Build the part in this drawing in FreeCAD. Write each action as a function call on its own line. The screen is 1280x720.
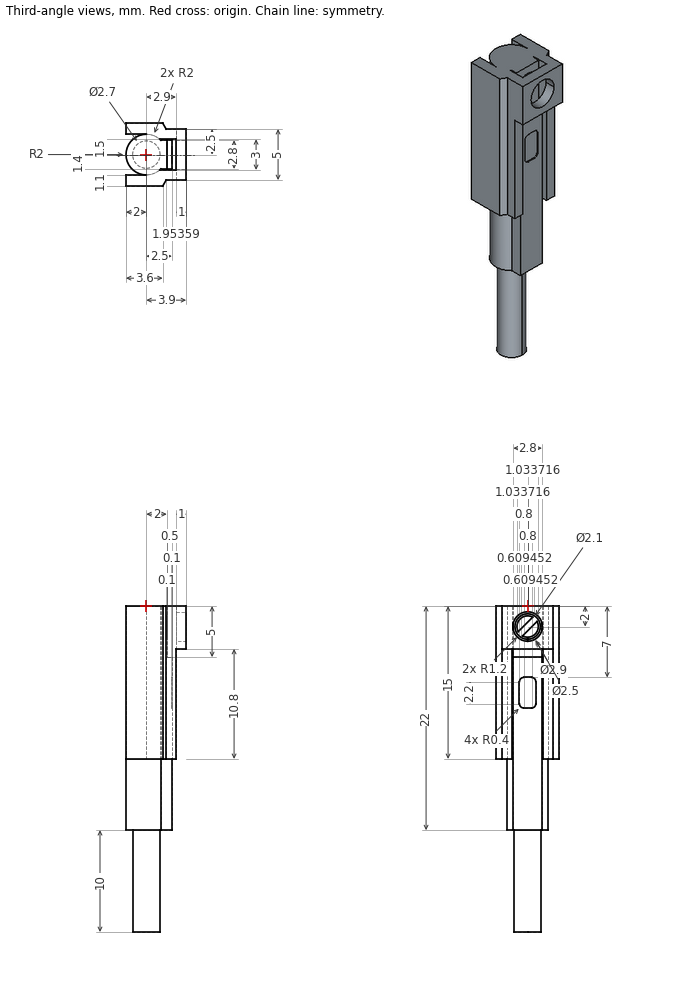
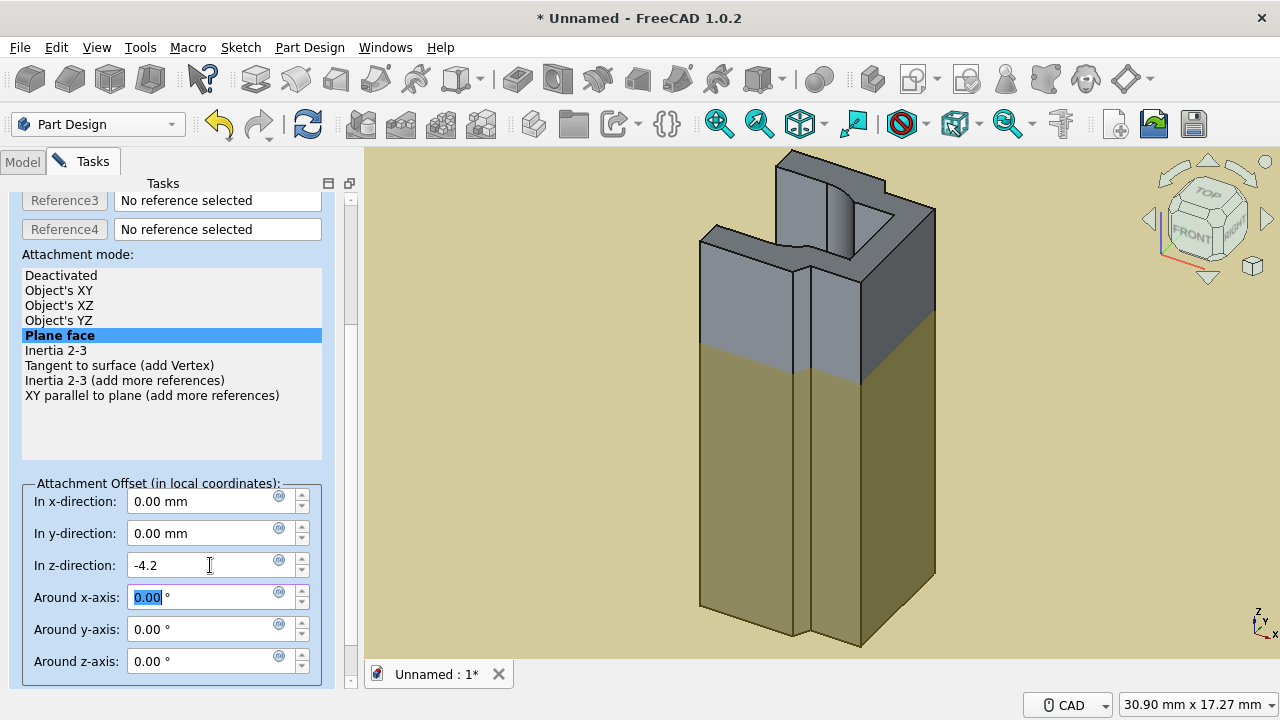
scroll(351, 440, up, 4)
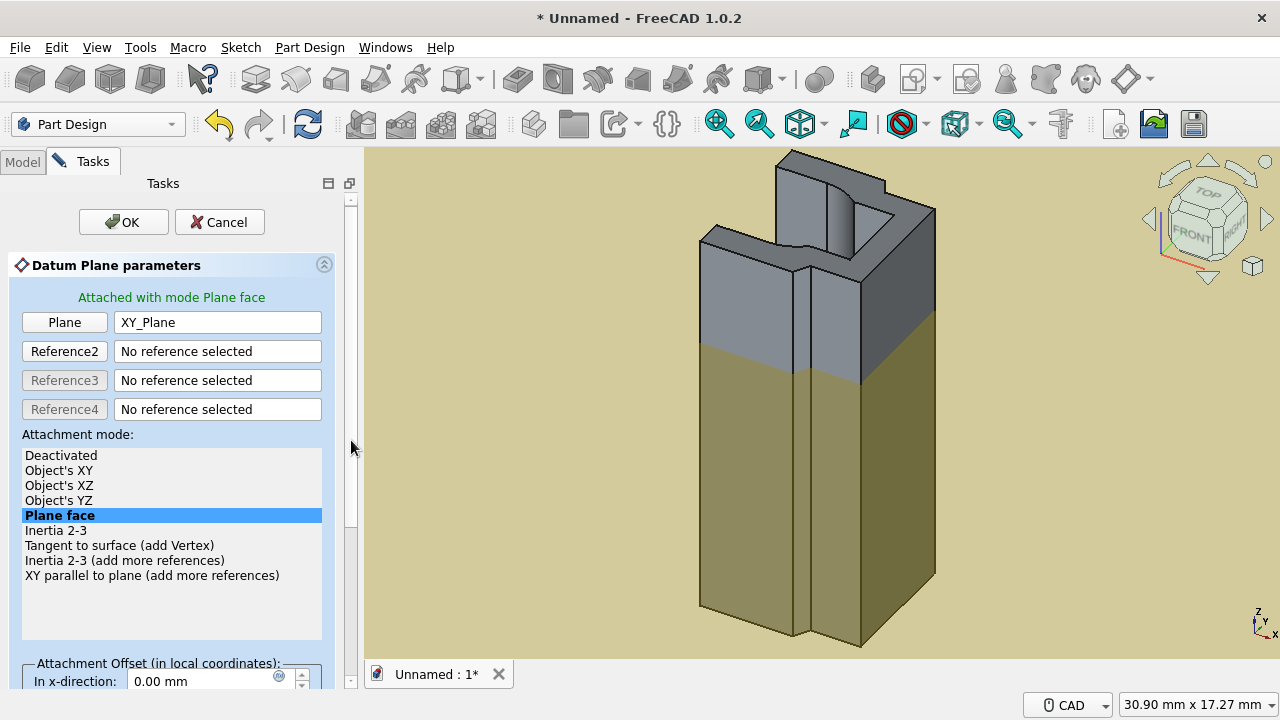
click(124, 222)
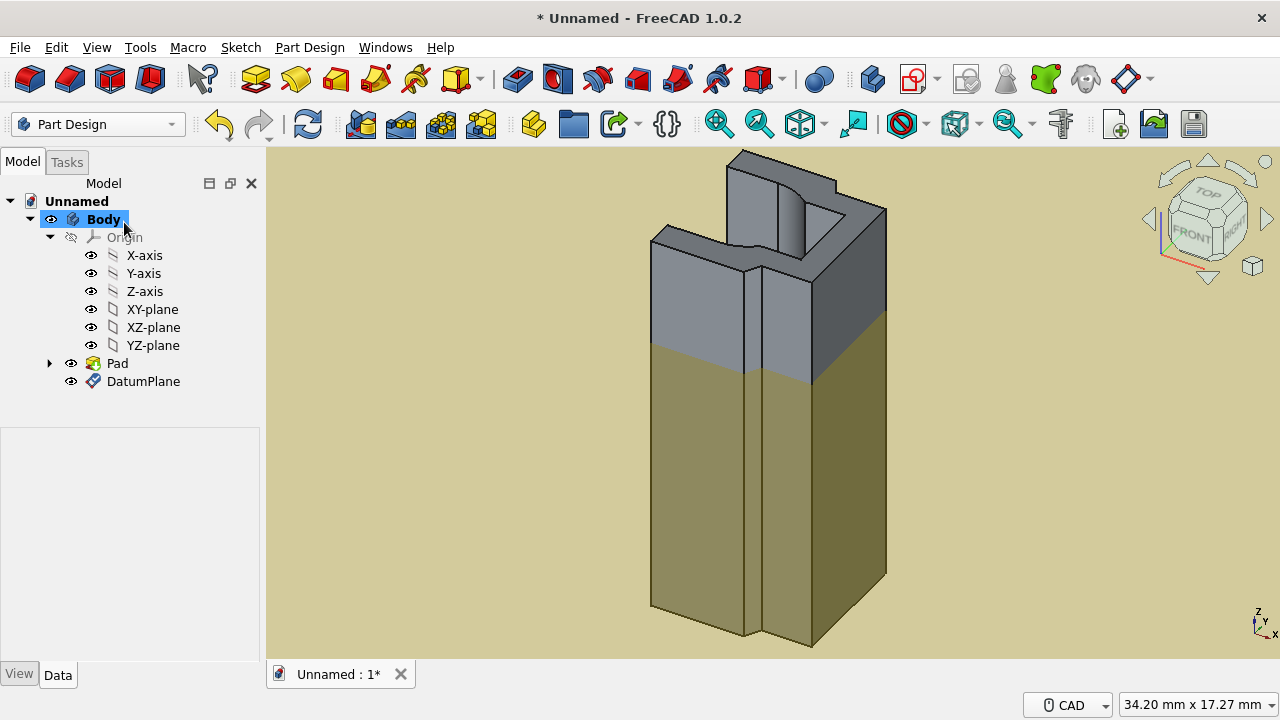
click(116, 381)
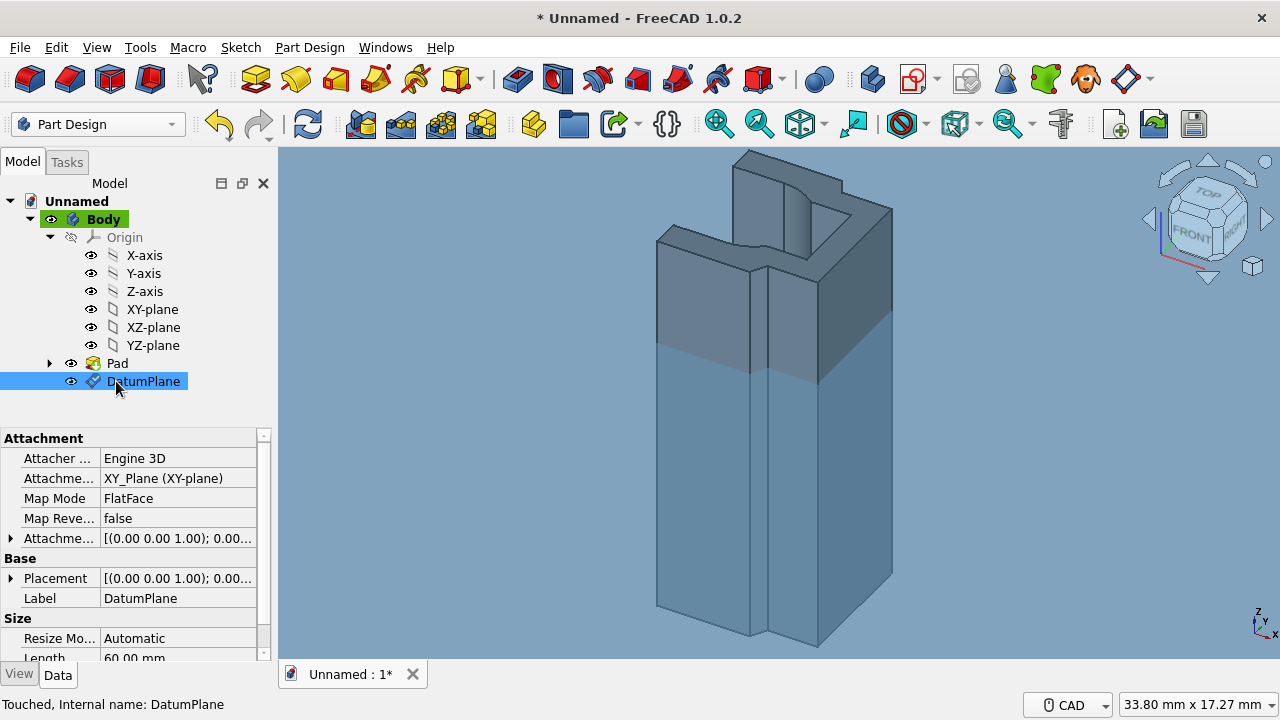
click(914, 80)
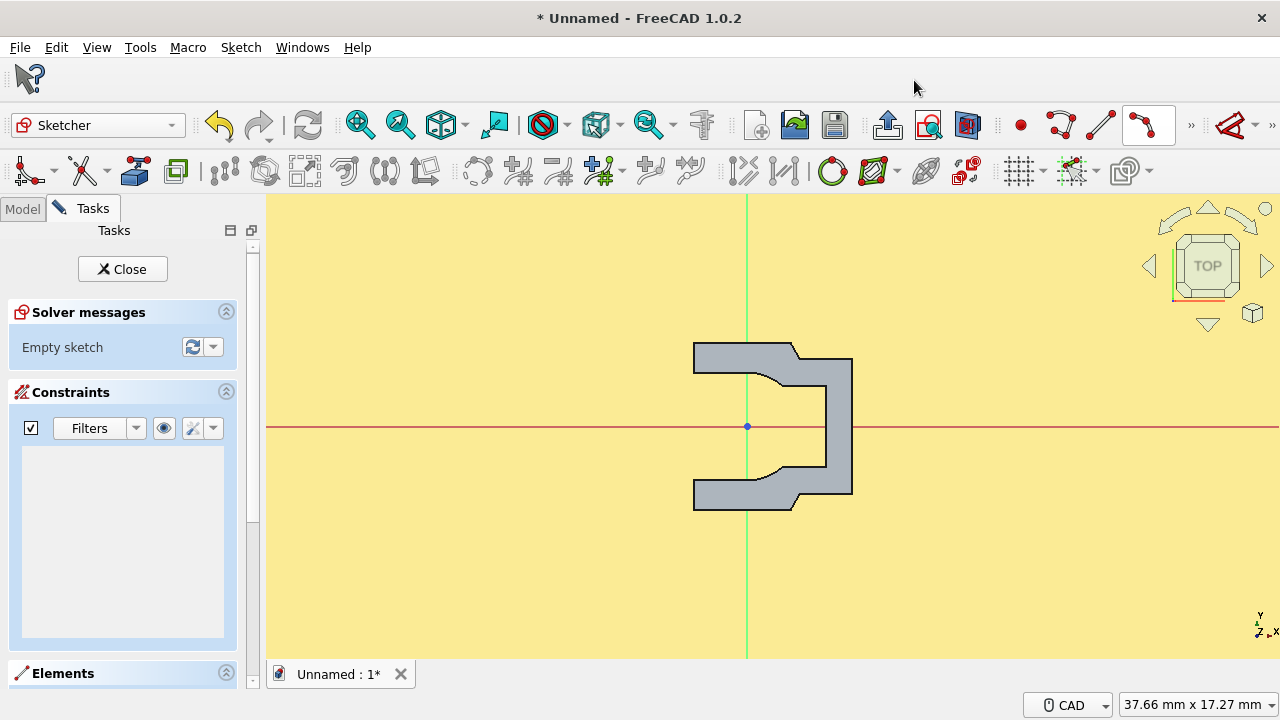
click(968, 126)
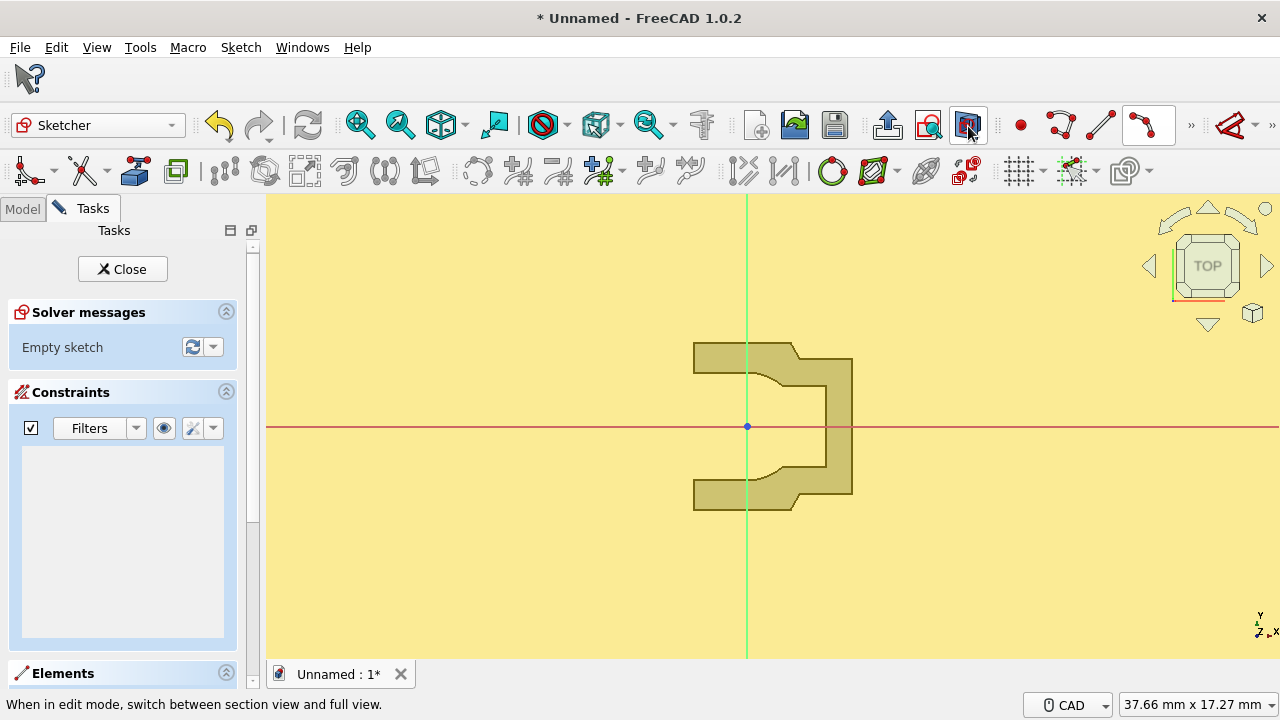
scroll(878, 426, up, 4)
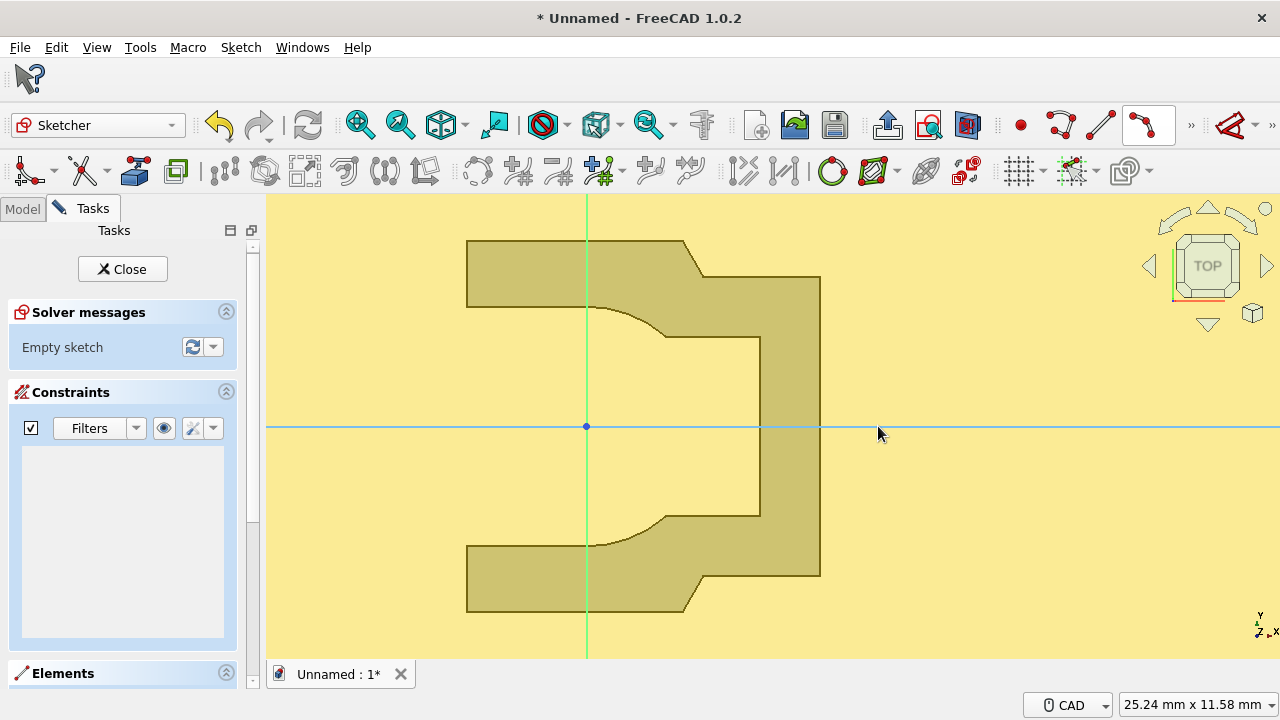
key(g)
key(r)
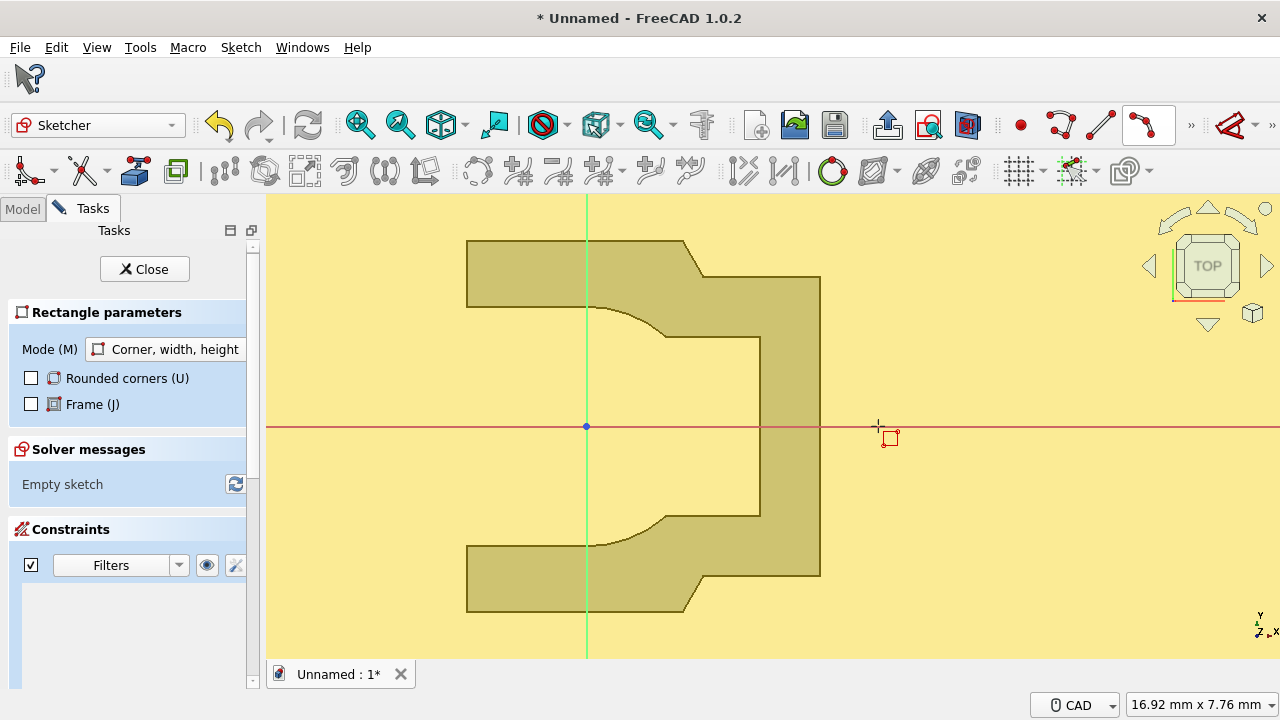
click(760, 277)
click(820, 576)
key(Escape)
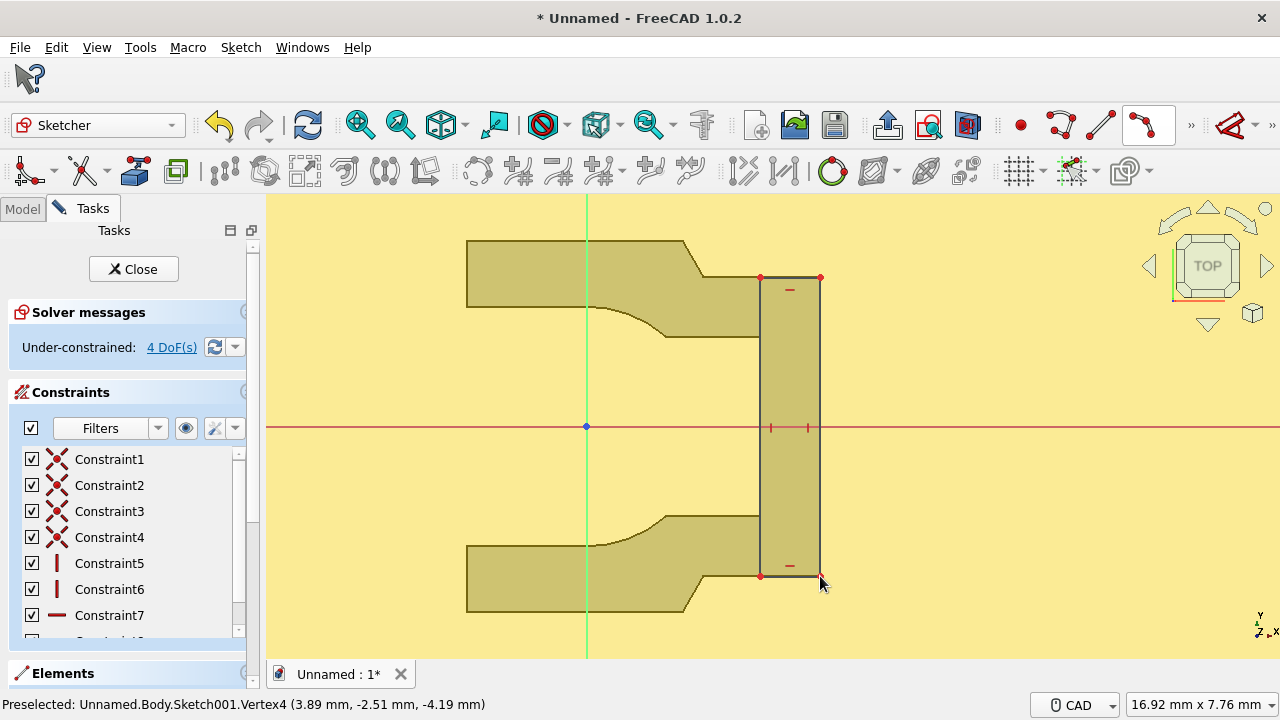
click(1230, 126)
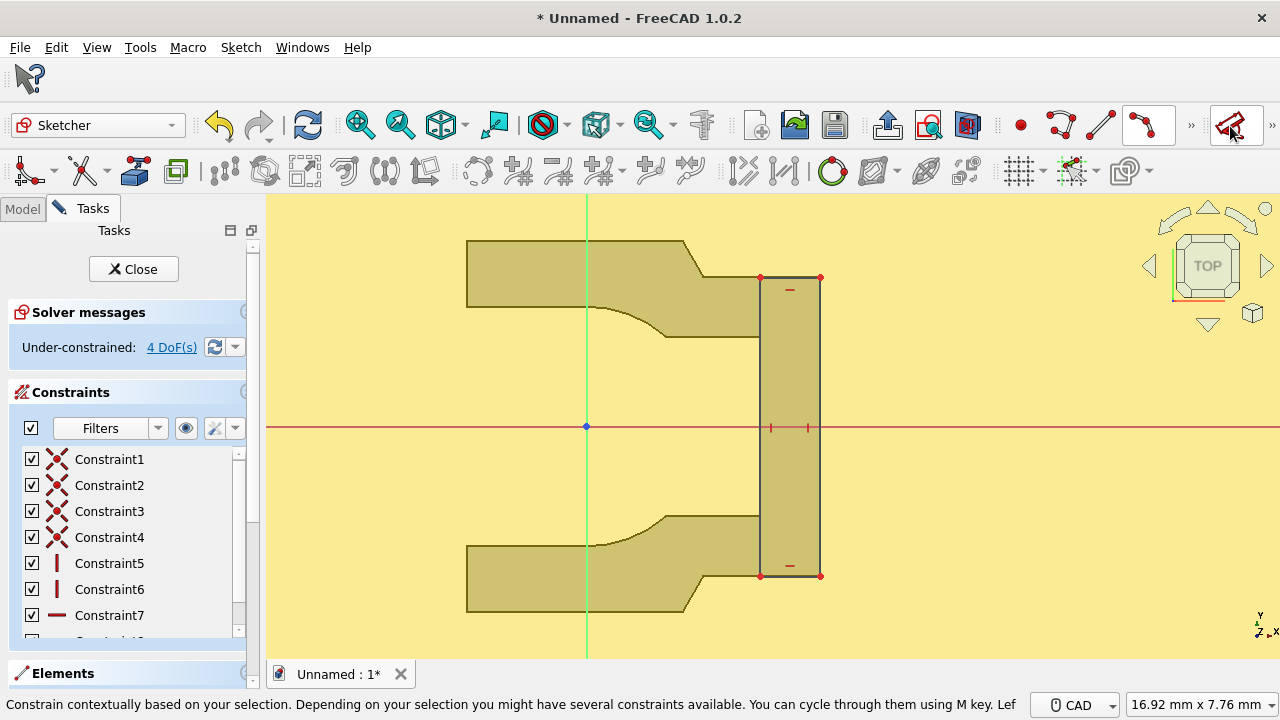
click(760, 368)
click(794, 359)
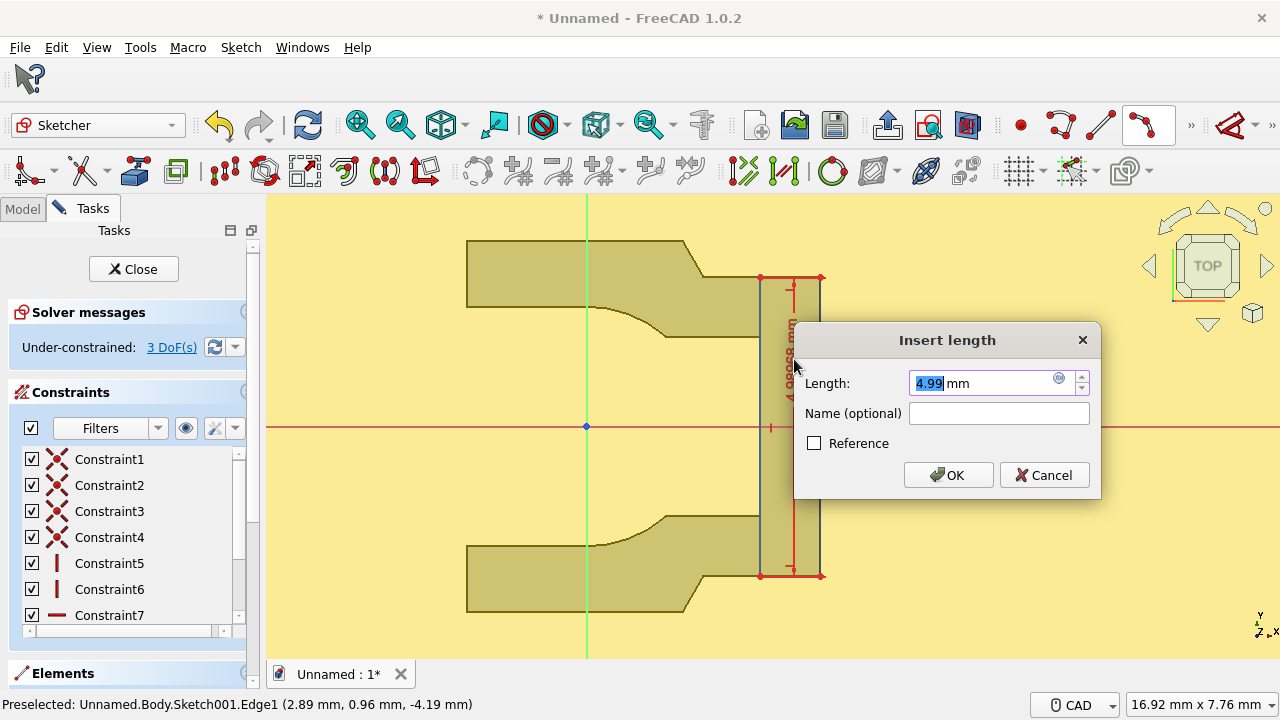
text(5)
key(Return)